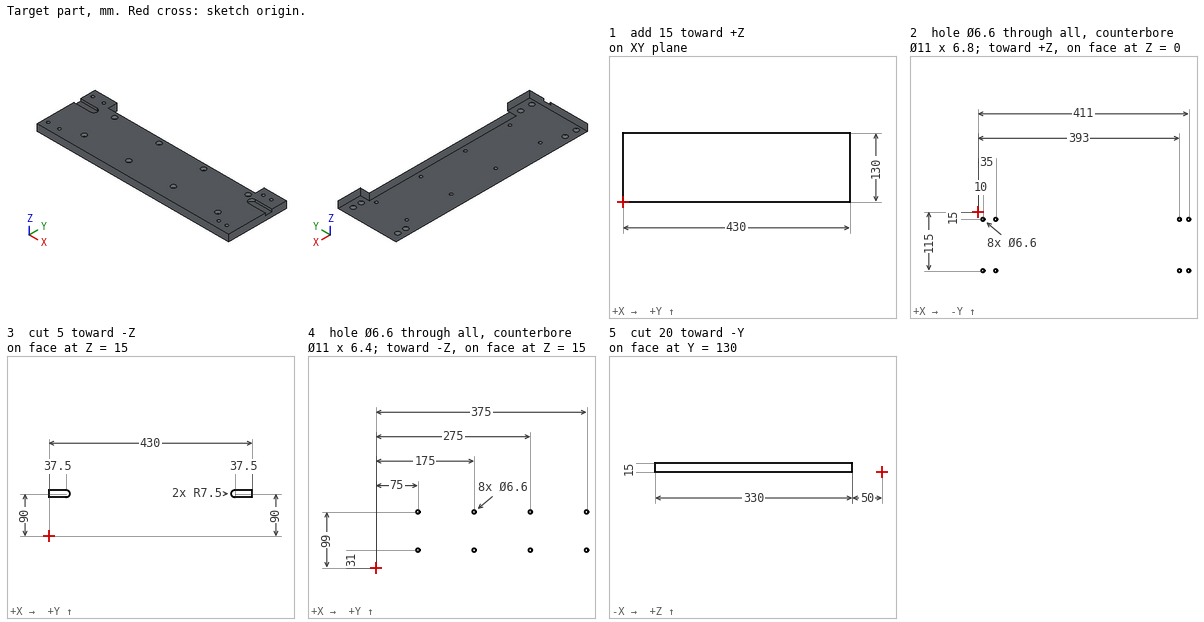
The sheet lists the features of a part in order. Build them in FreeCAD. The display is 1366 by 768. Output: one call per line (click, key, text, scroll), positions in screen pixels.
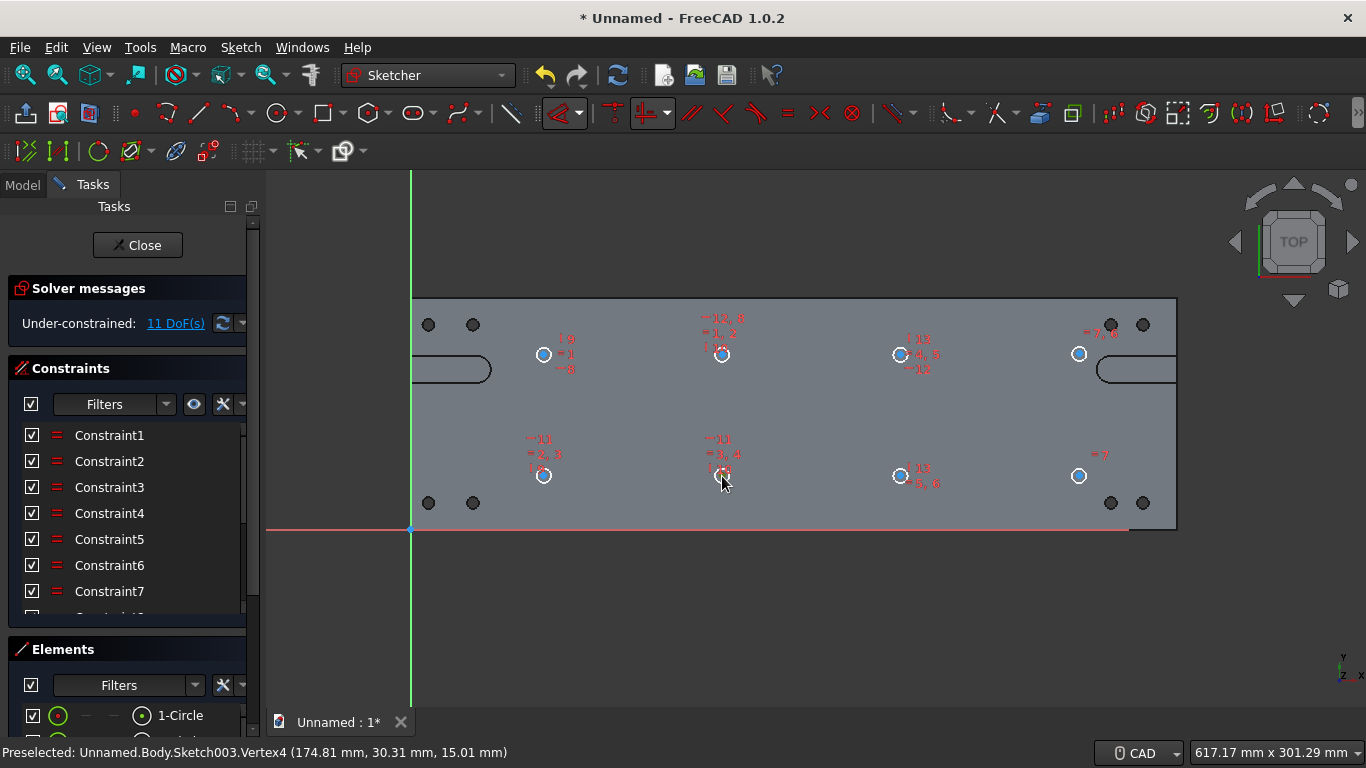
click(900, 476)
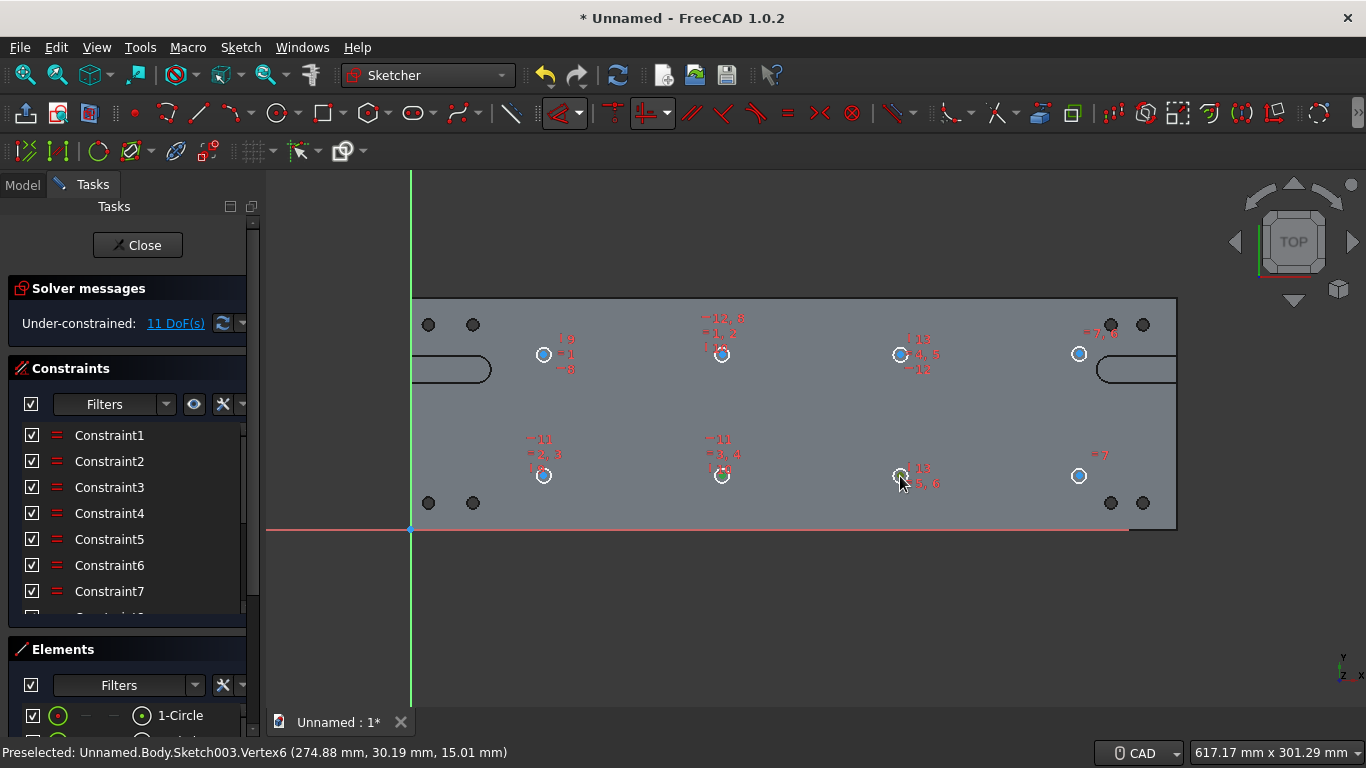
click(670, 114)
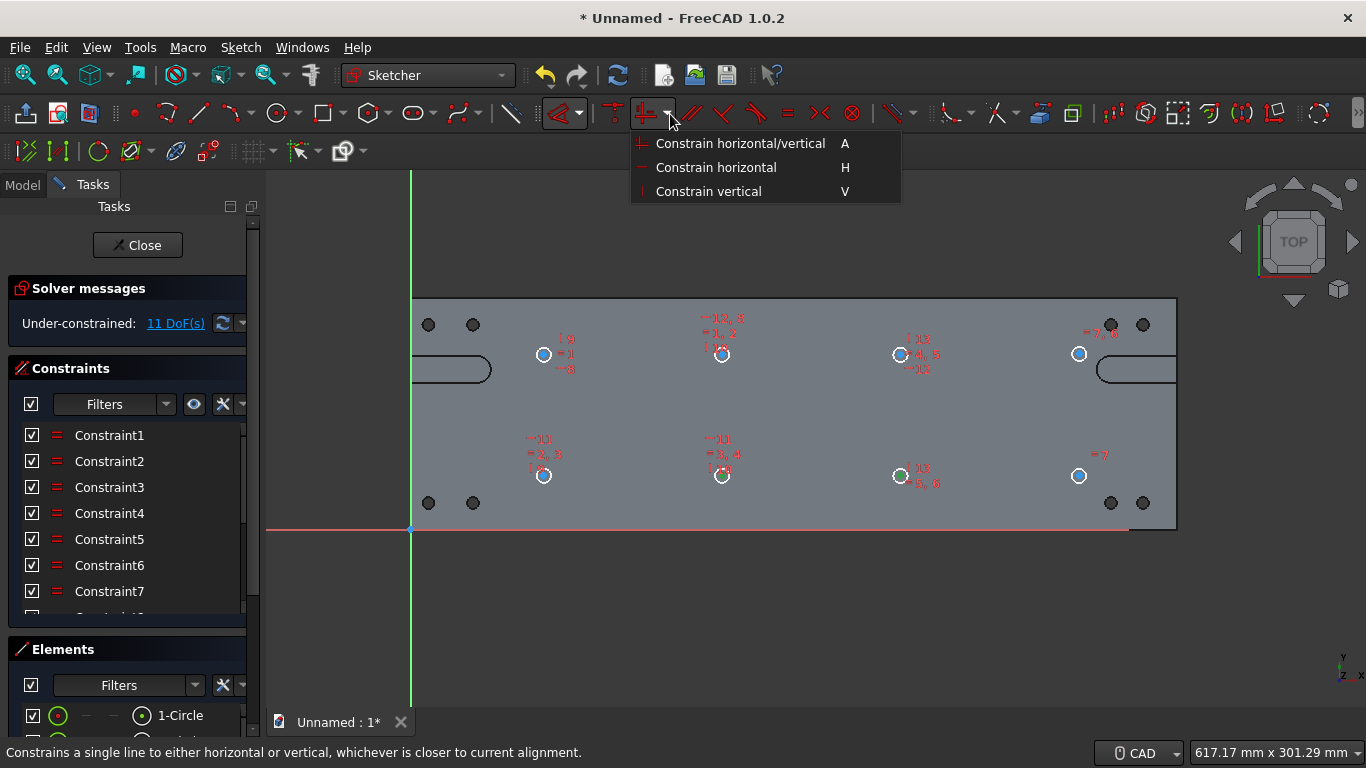
click(766, 167)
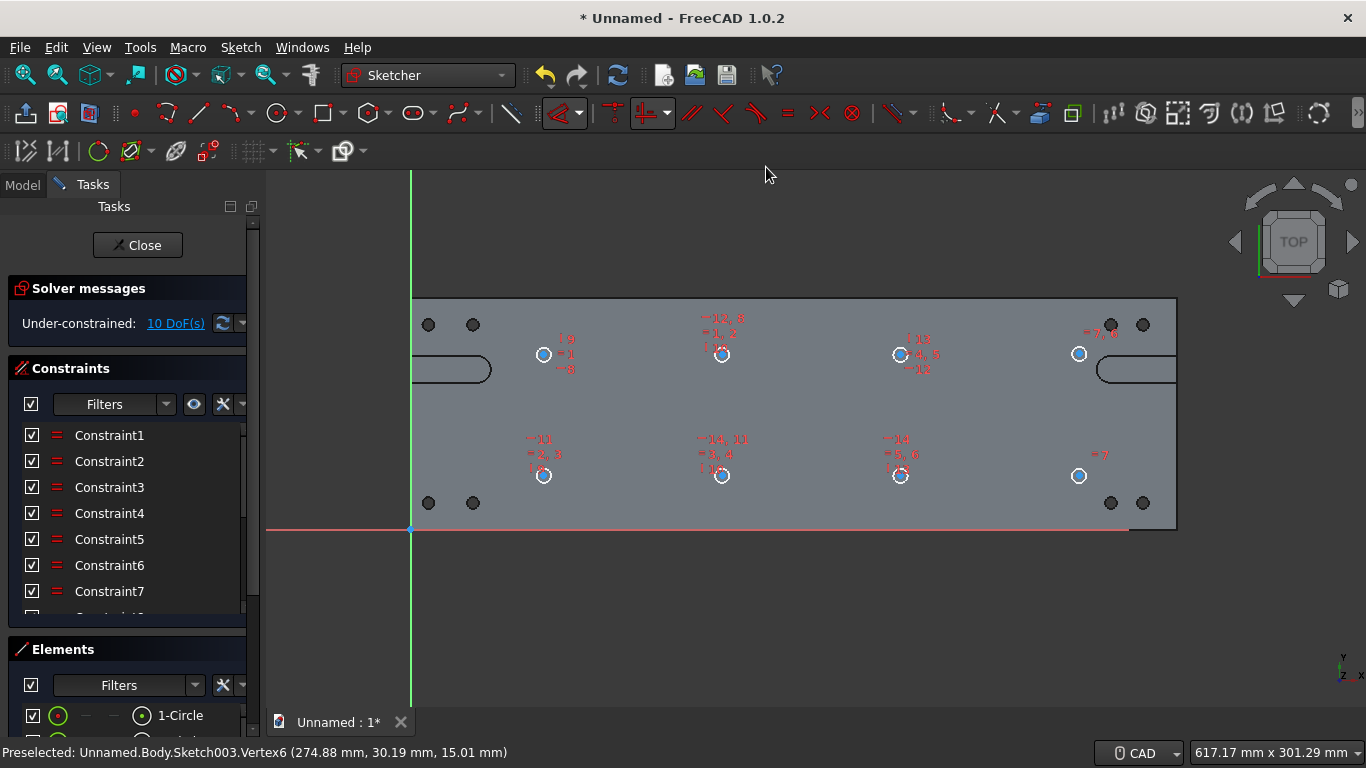
click(900, 355)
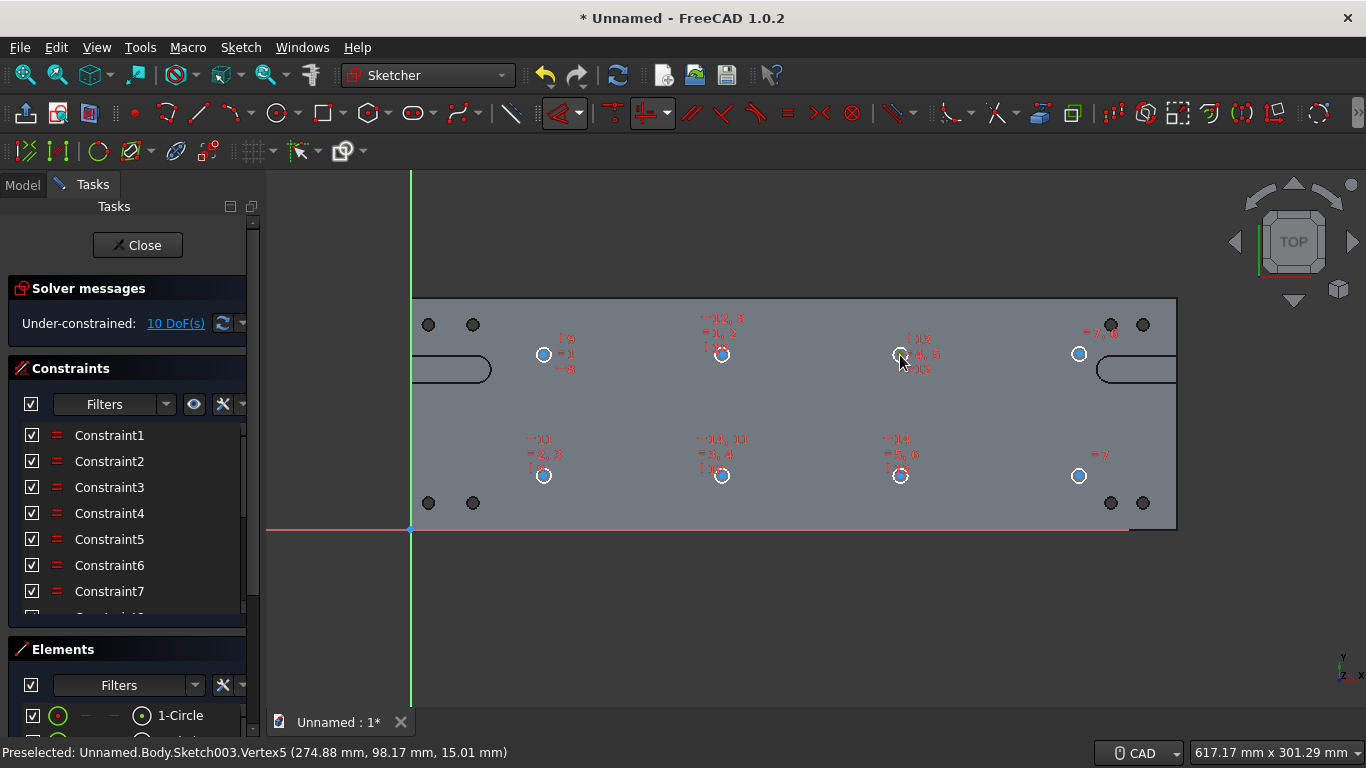
click(1079, 354)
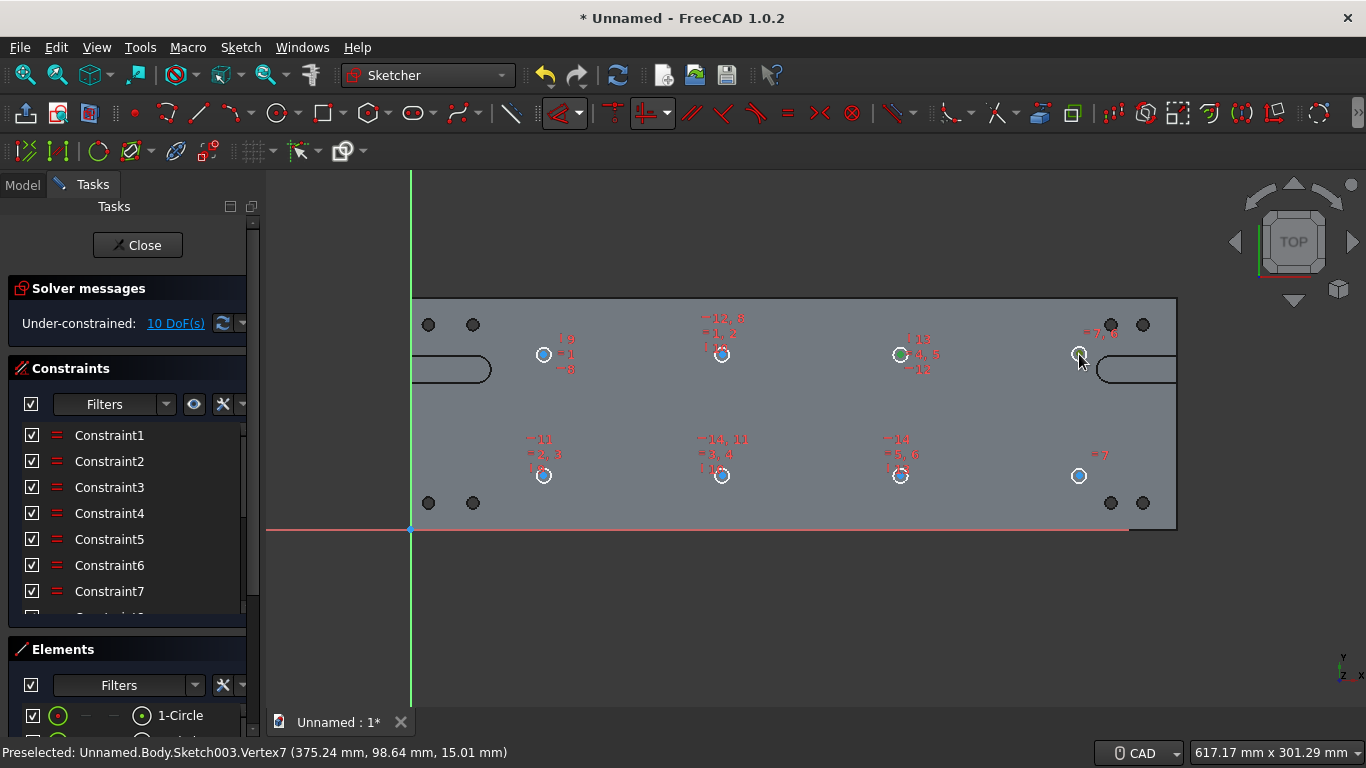
click(670, 114)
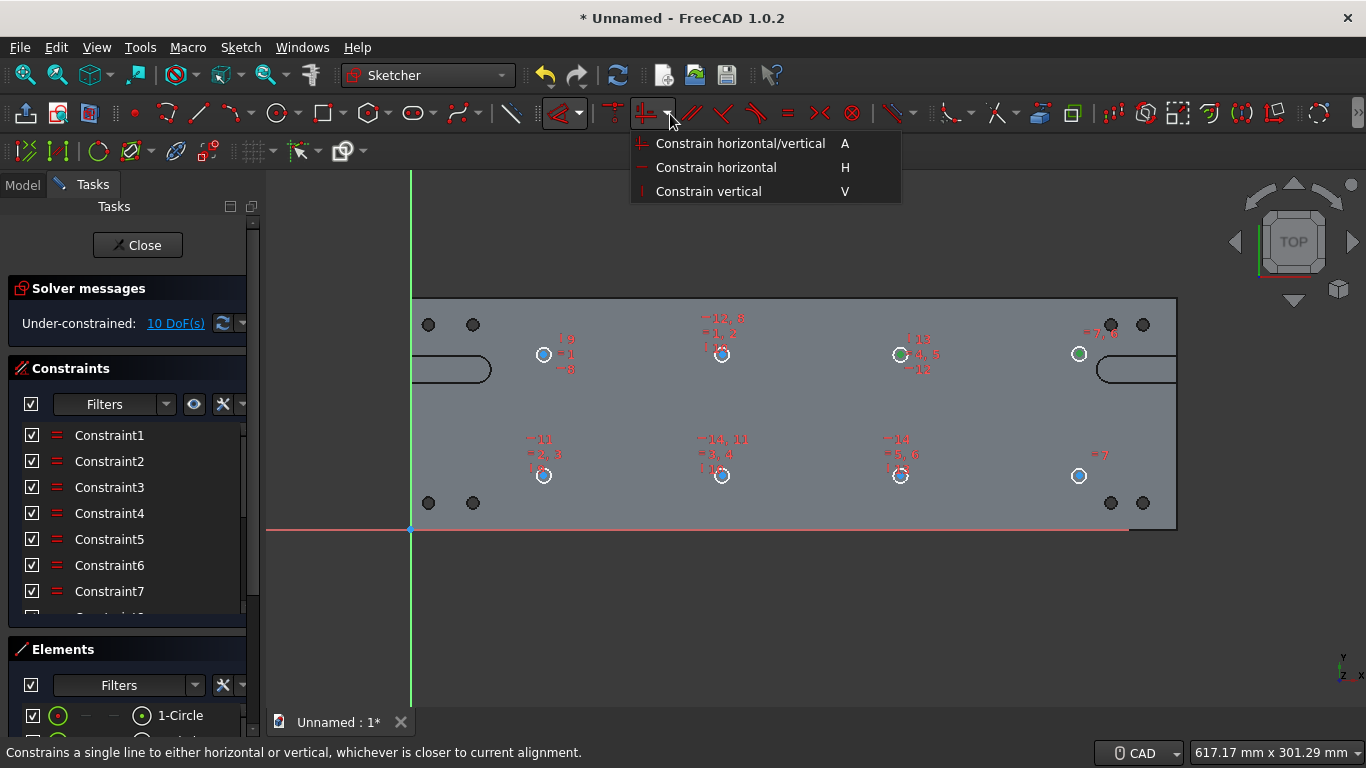
click(766, 167)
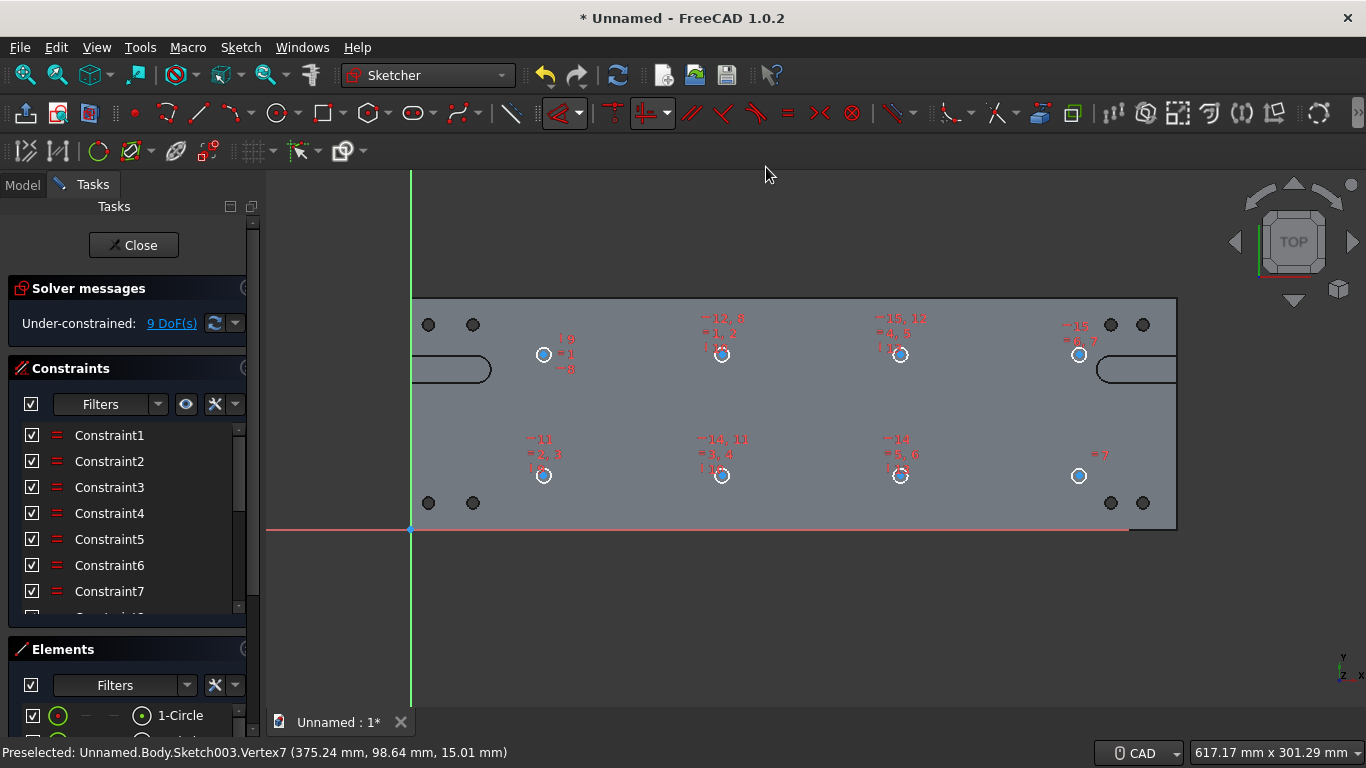
click(1079, 355)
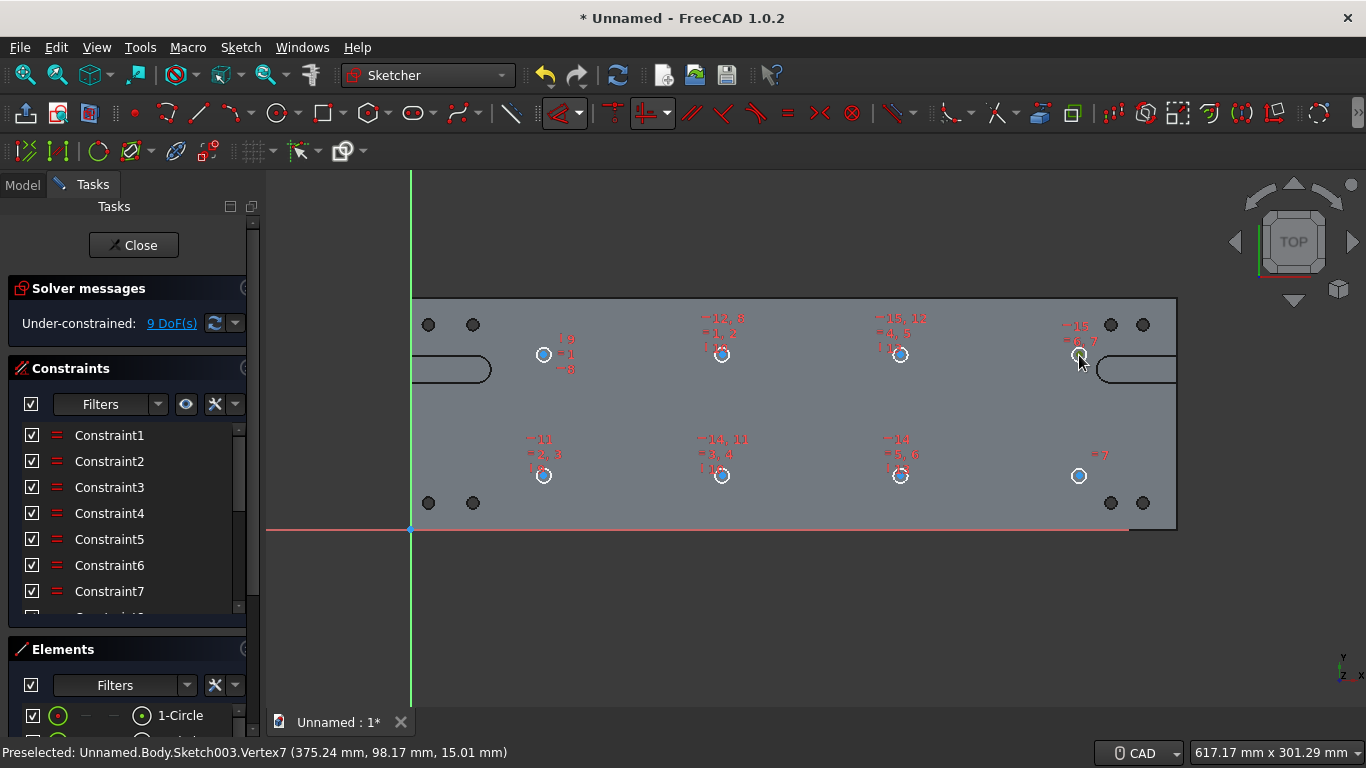
click(1079, 476)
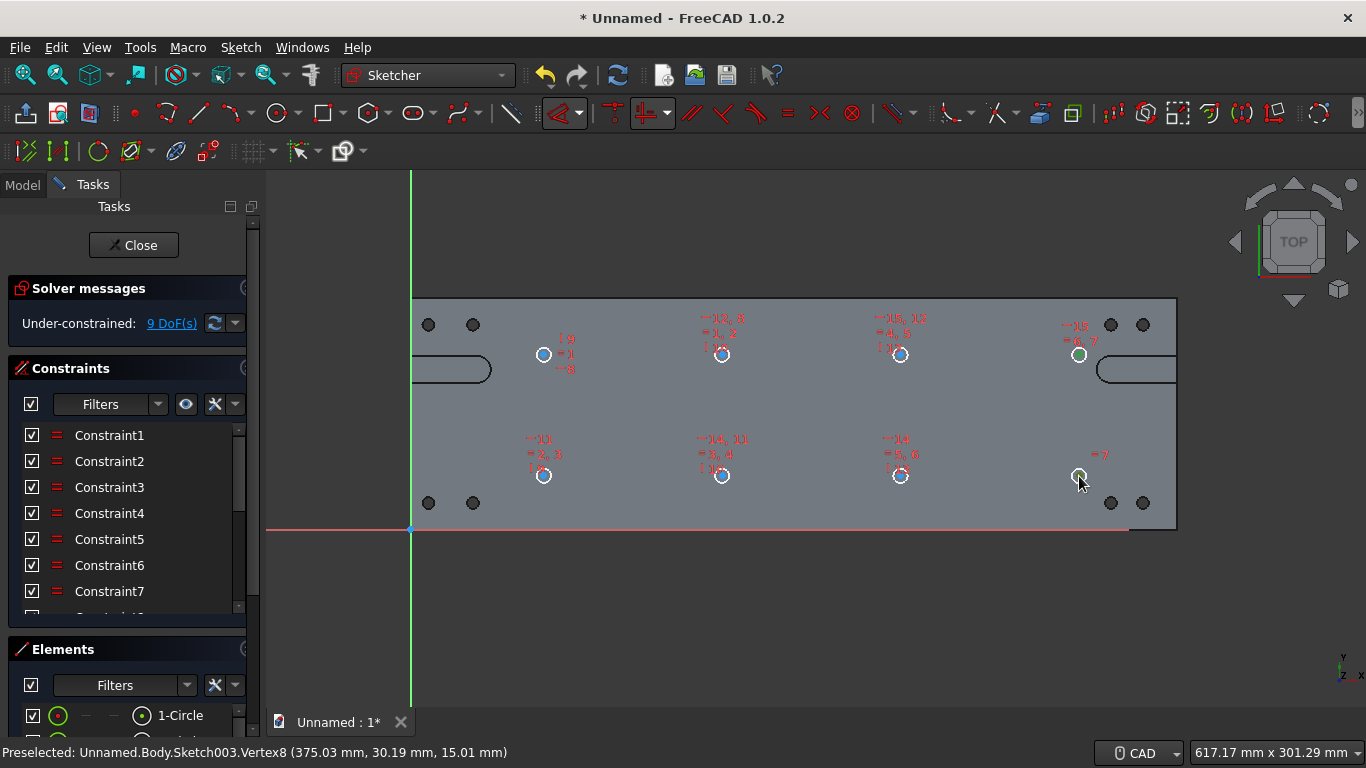
click(670, 114)